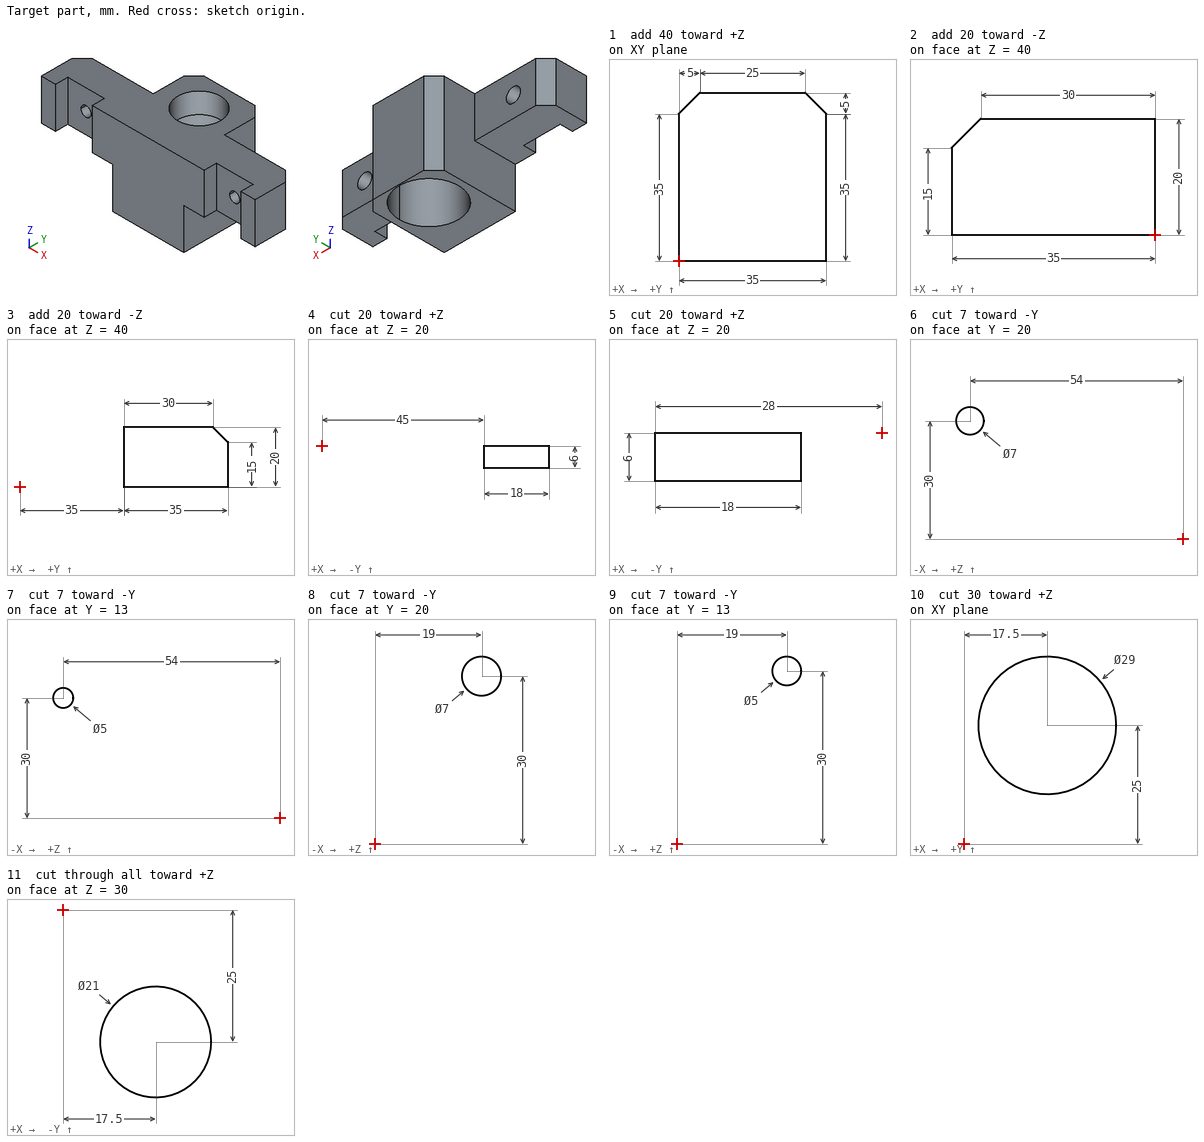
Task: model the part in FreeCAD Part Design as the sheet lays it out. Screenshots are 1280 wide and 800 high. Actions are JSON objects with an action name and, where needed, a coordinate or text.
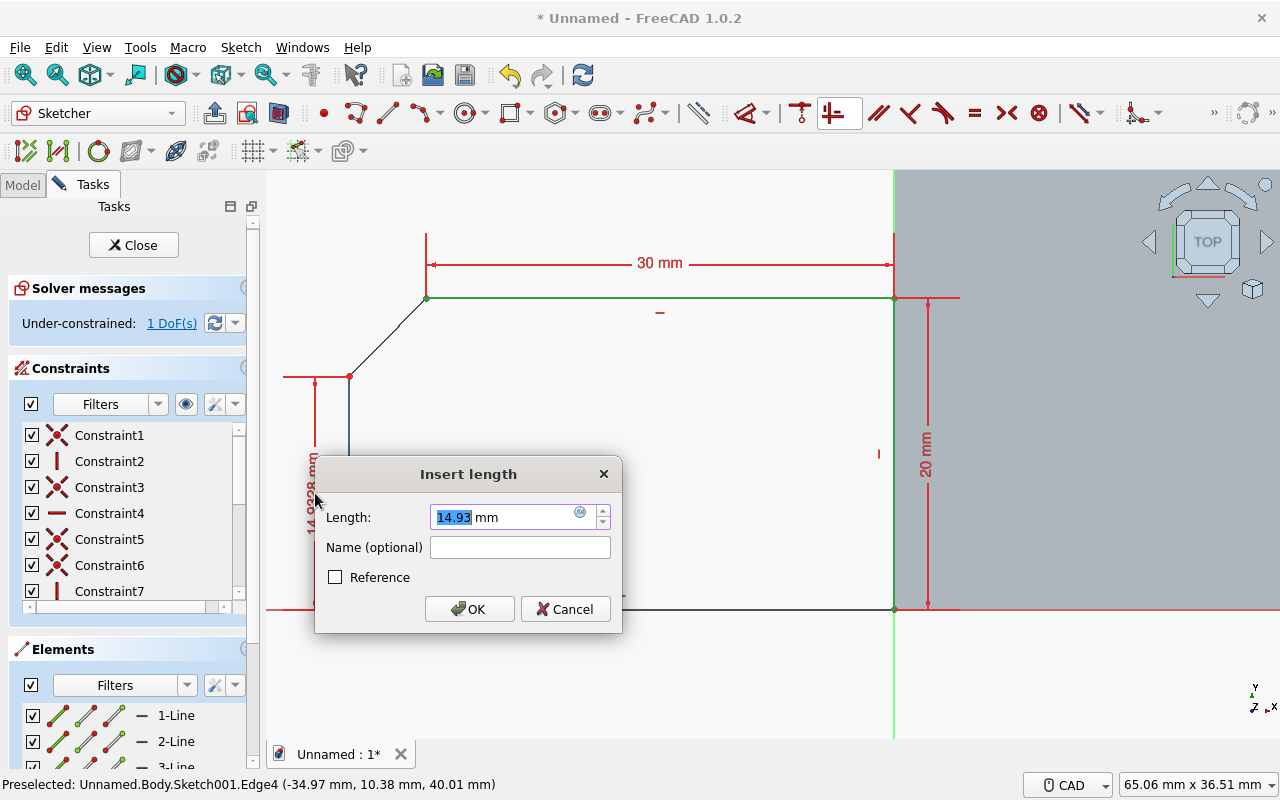
{"action": "type", "text": "15"}
{"action": "key", "text": "Return"}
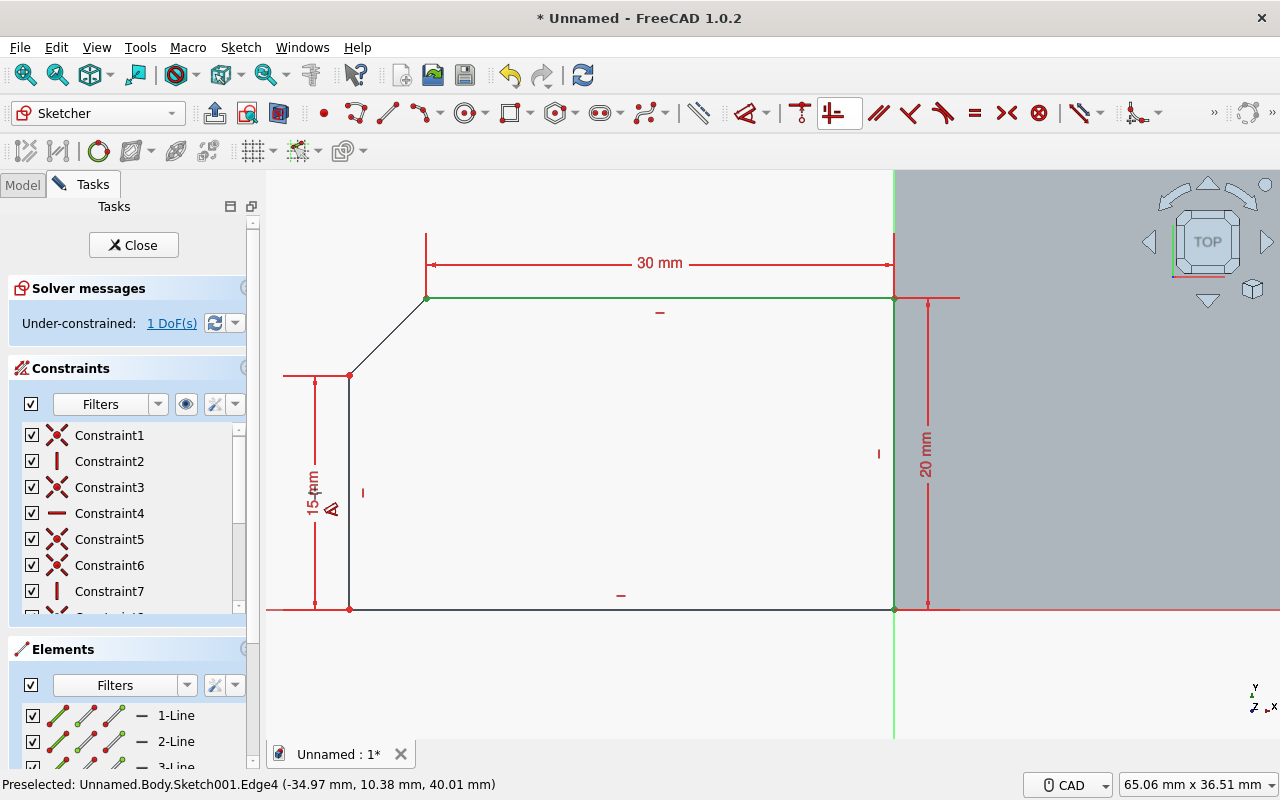
{"action": "left_click", "coordinate": [513, 610]}
{"action": "left_click", "coordinate": [622, 644]}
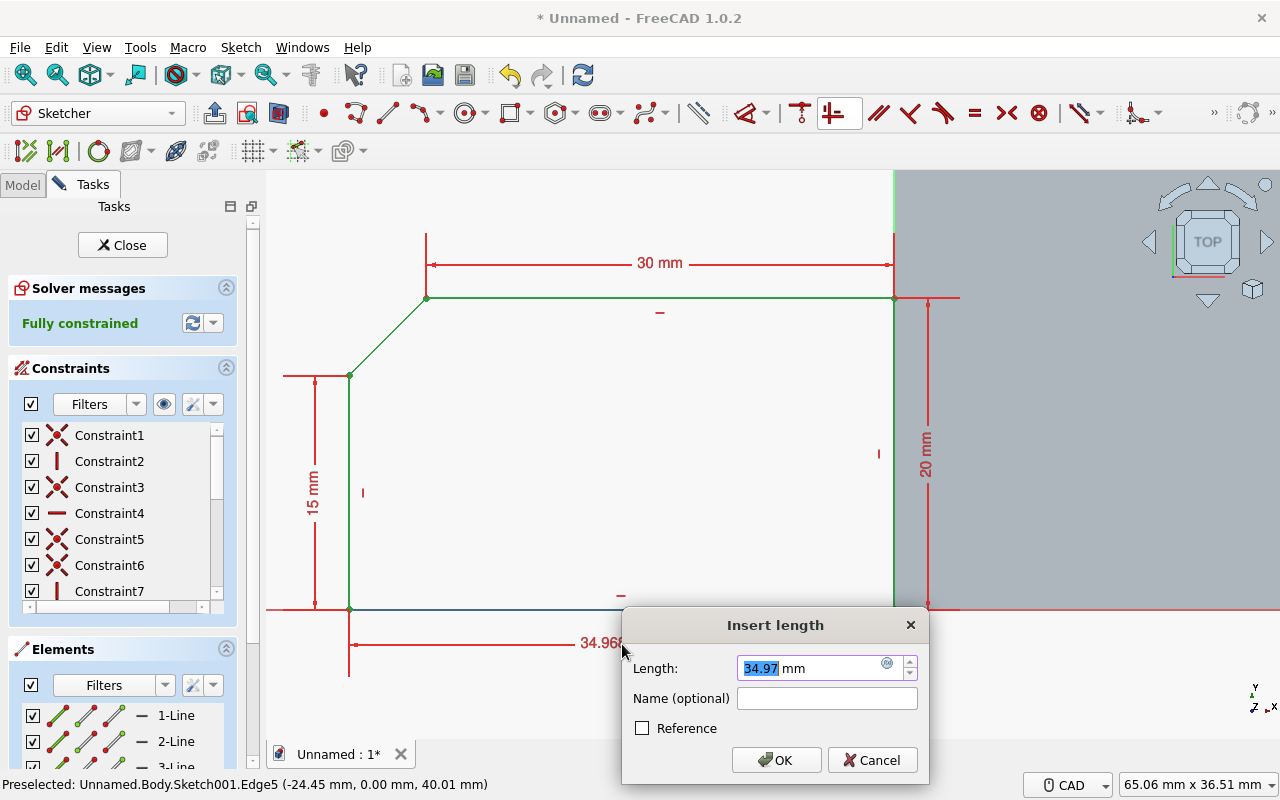
{"action": "type", "text": "35"}
{"action": "key", "text": "Return"}
{"action": "key", "text": "Escape"}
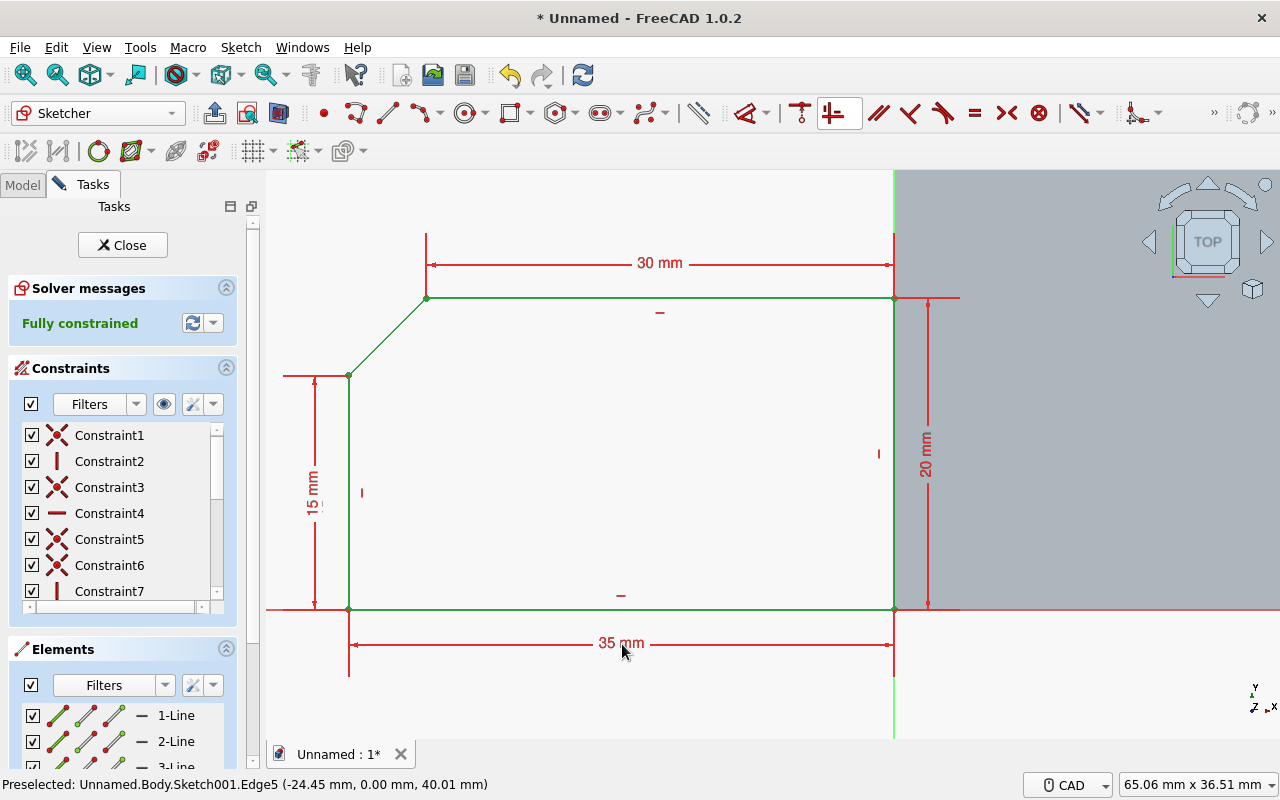
{"action": "left_click", "coordinate": [123, 245]}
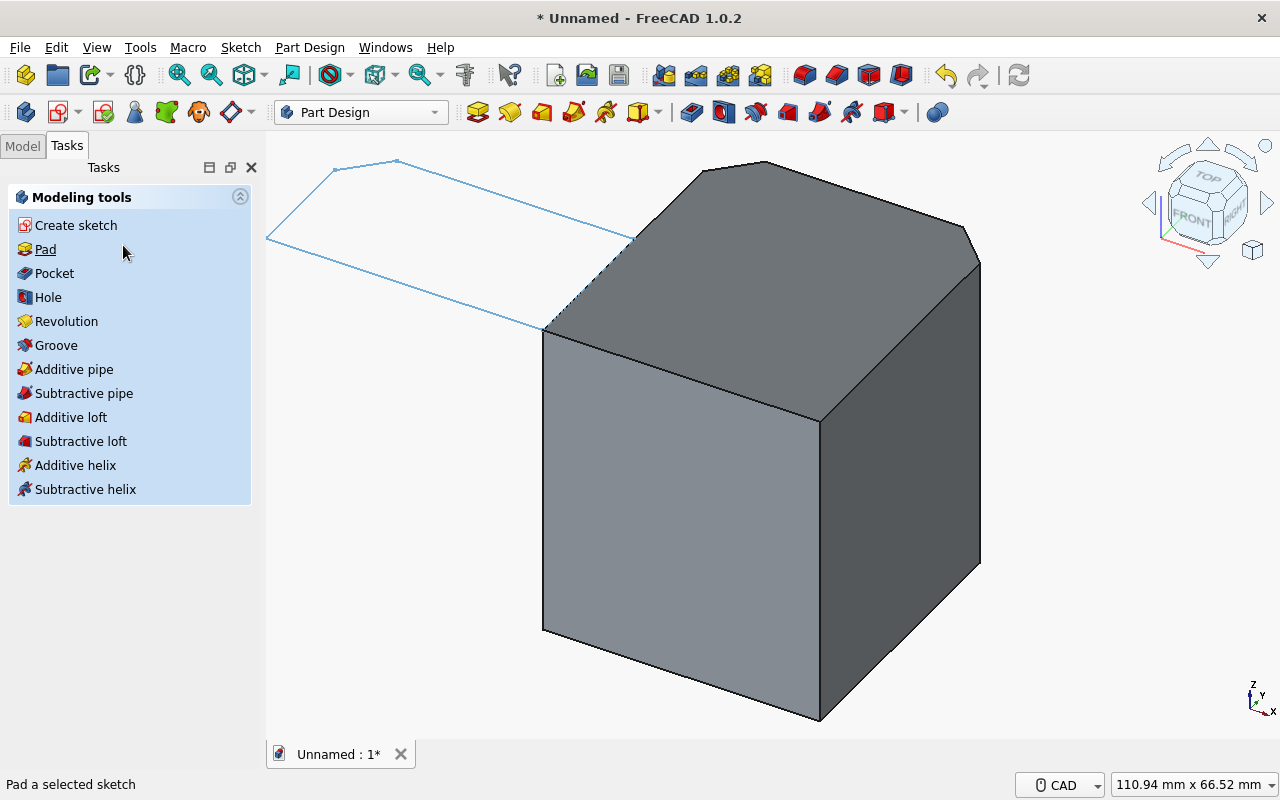
{"action": "left_click", "coordinate": [478, 112]}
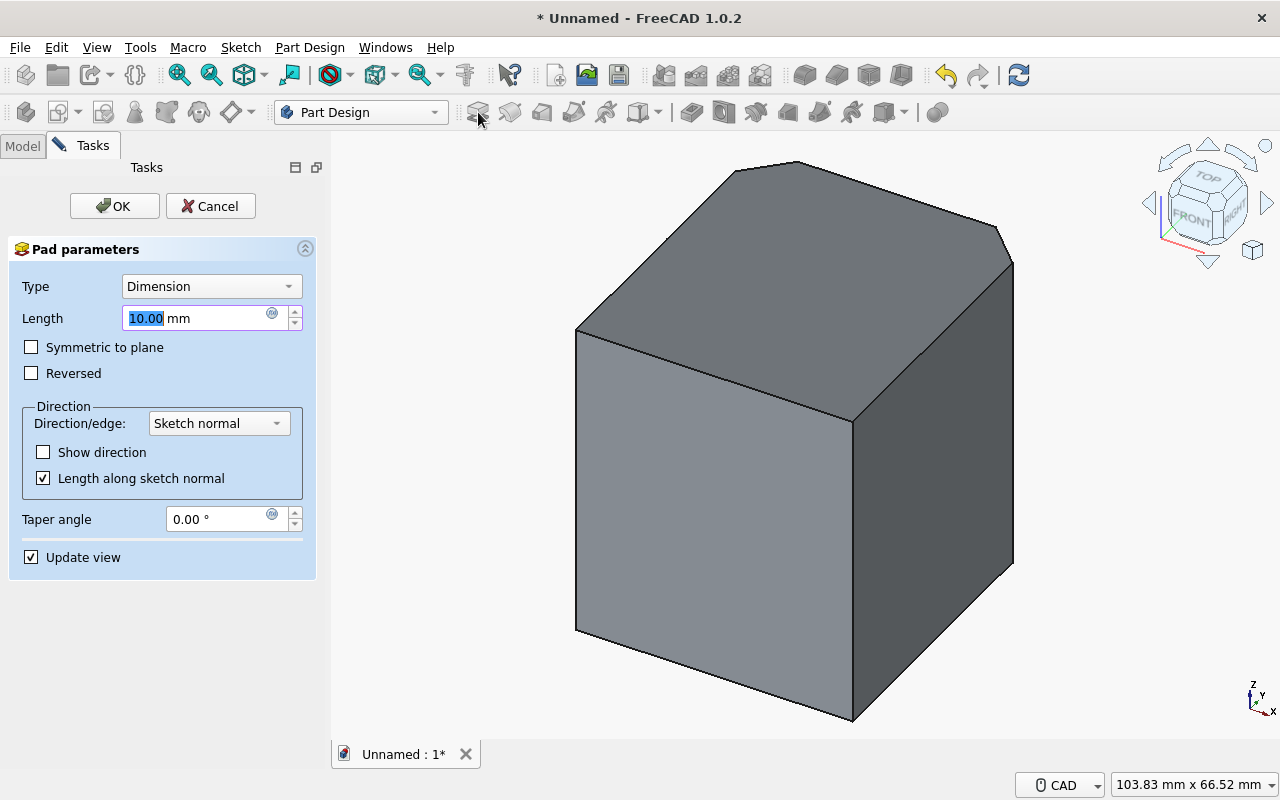
{"action": "type", "text": "20"}
{"action": "key", "text": "Tab"}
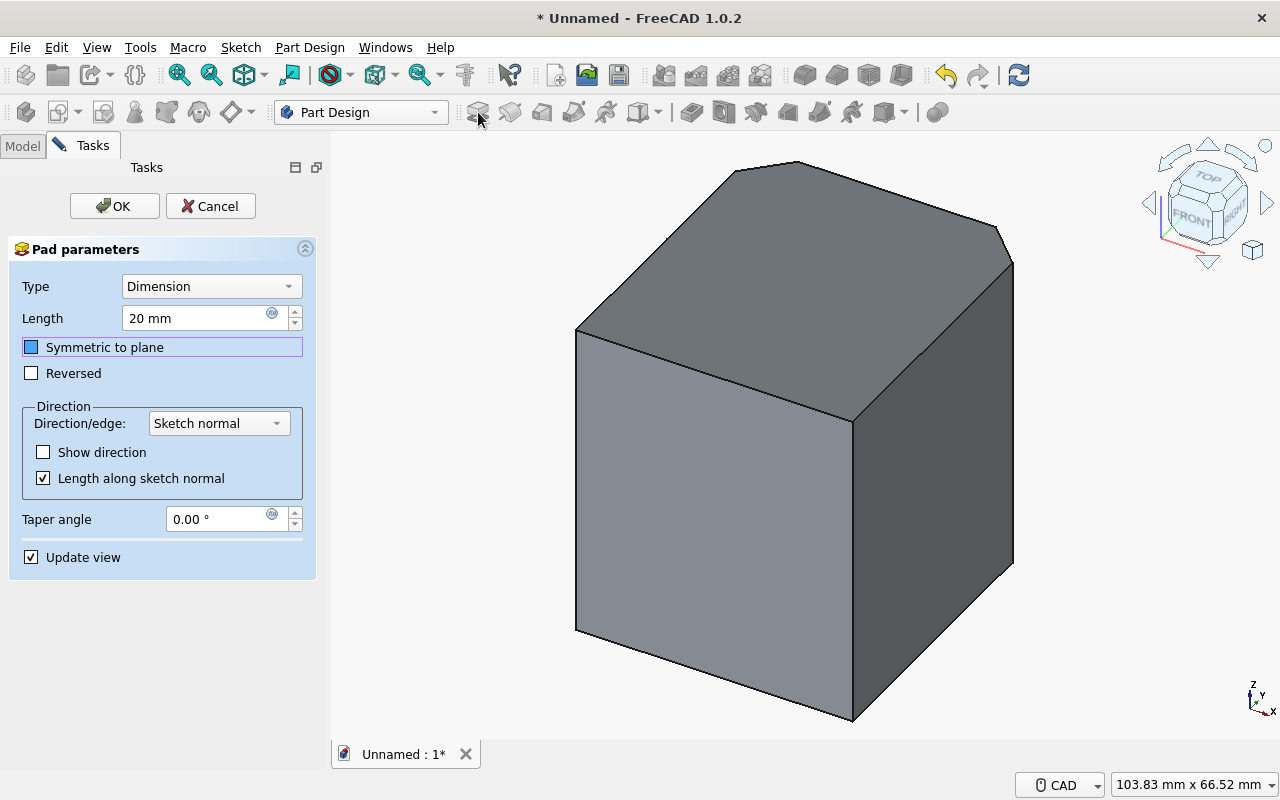
{"action": "left_click", "coordinate": [30, 373]}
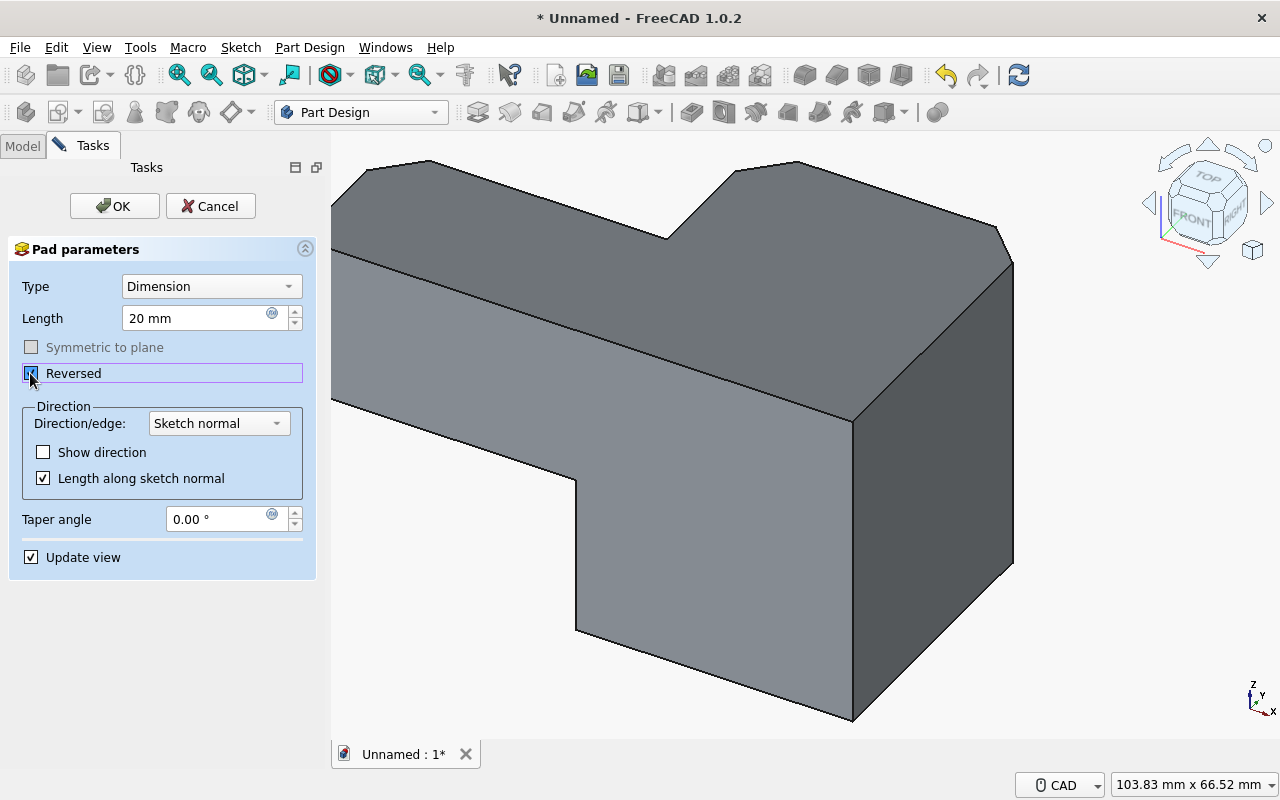
{"action": "left_click", "coordinate": [115, 206]}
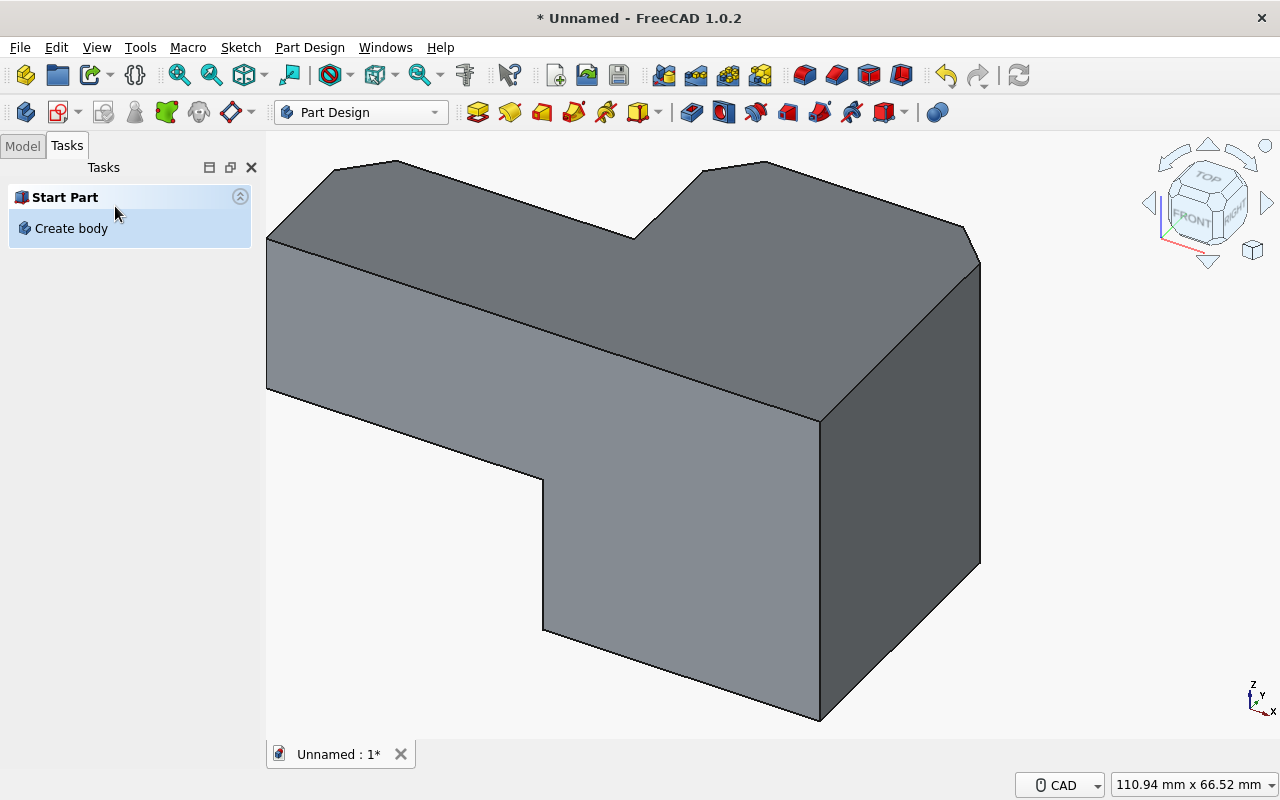
{"action": "left_click", "coordinate": [180, 76]}